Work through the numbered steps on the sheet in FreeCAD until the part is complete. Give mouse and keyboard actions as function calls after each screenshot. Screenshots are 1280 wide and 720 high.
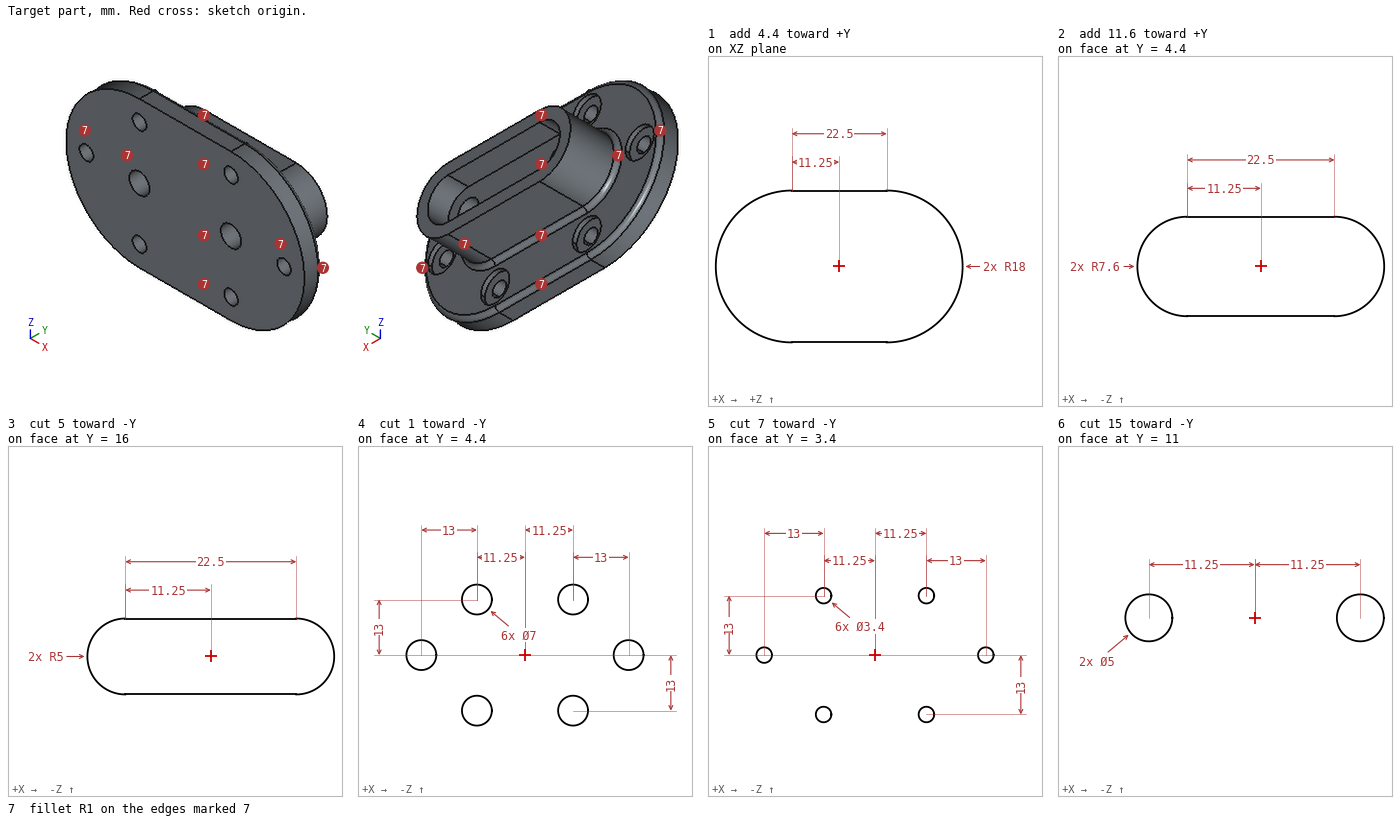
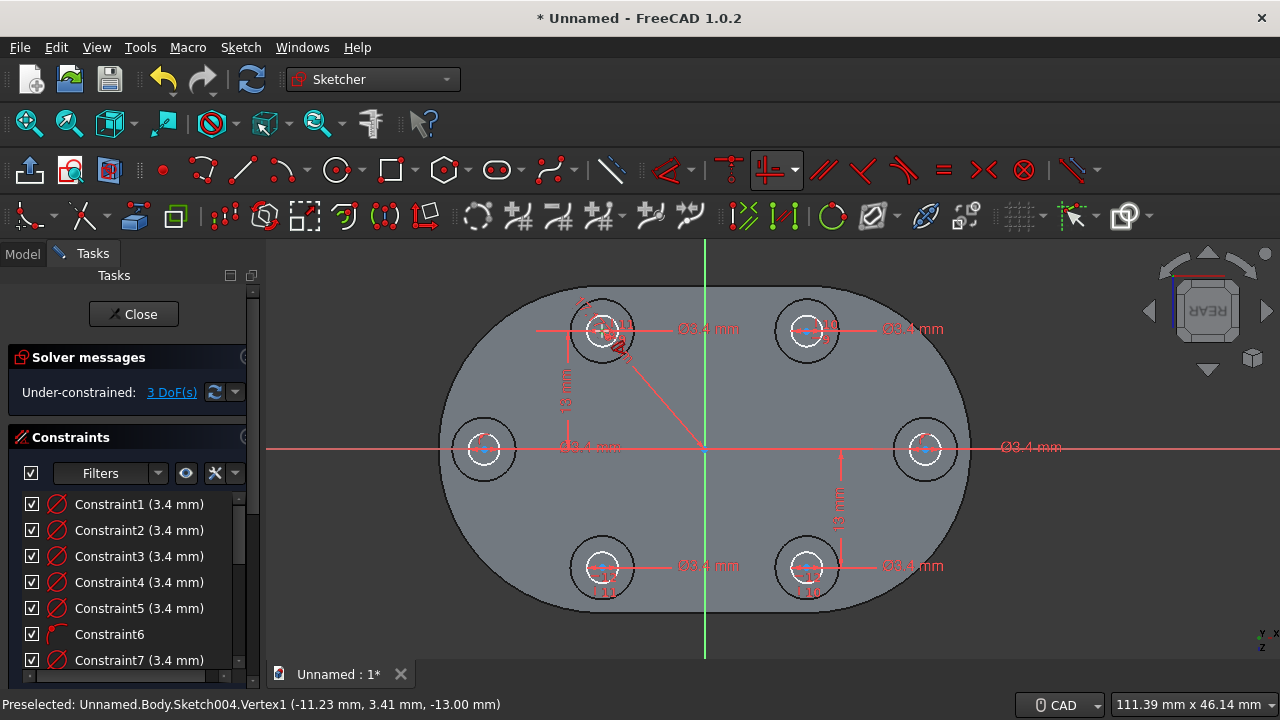
click(484, 449)
click(543, 297)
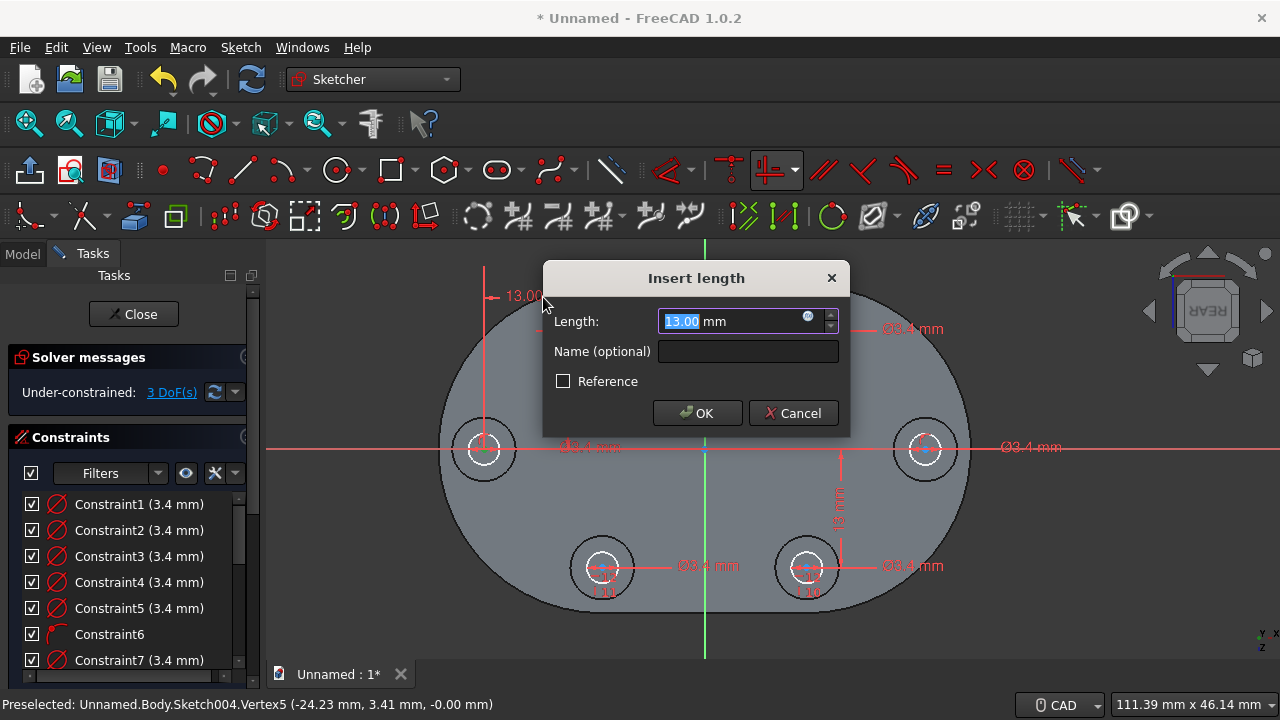
text(13)
key(Return)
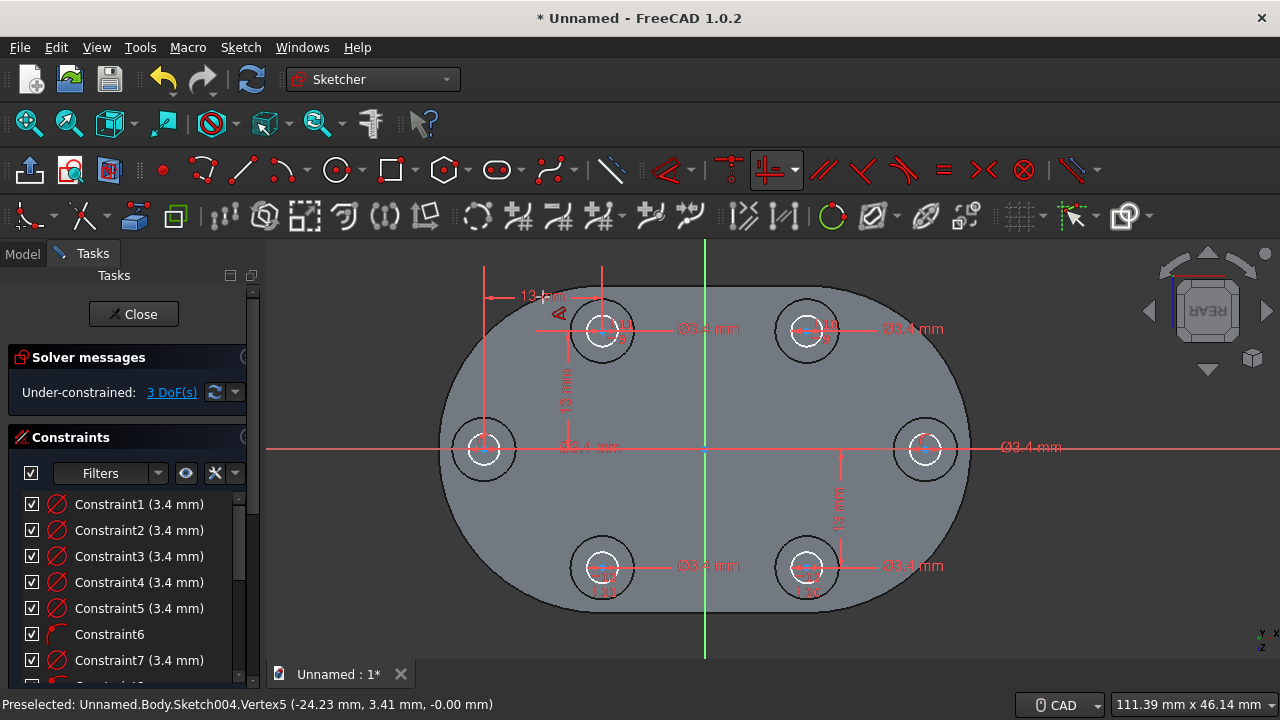
click(807, 331)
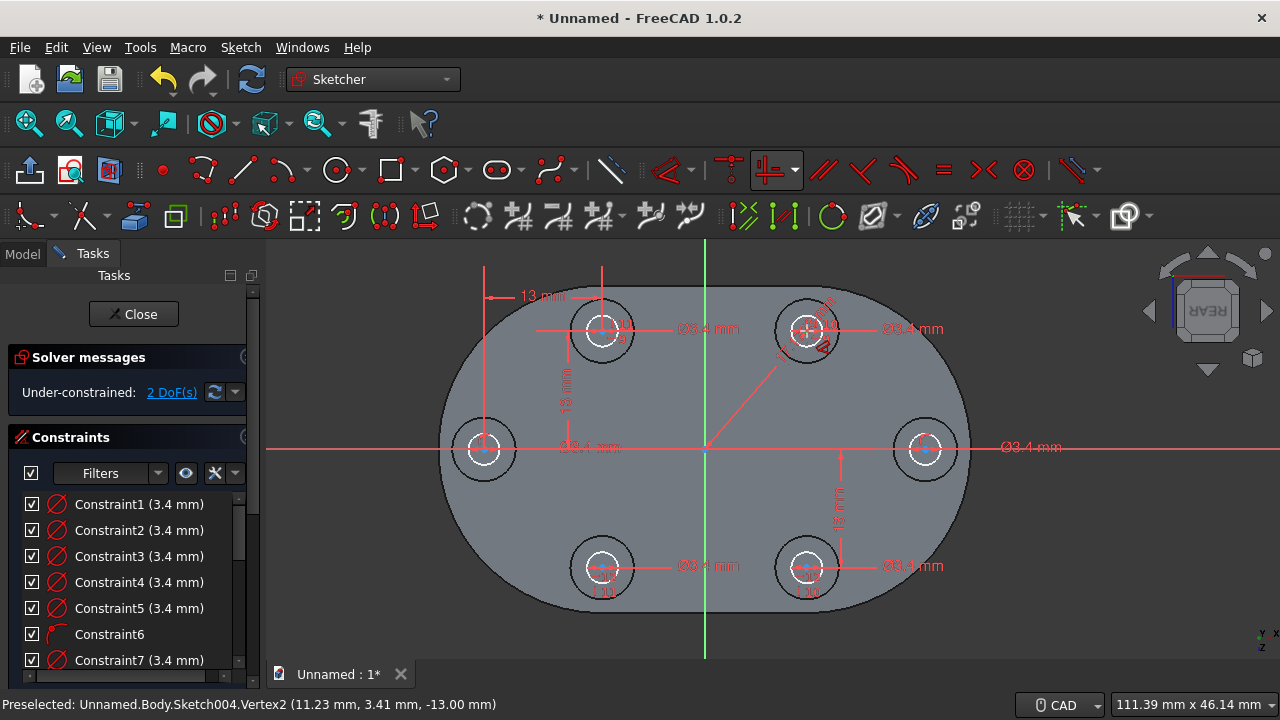
click(925, 449)
click(866, 297)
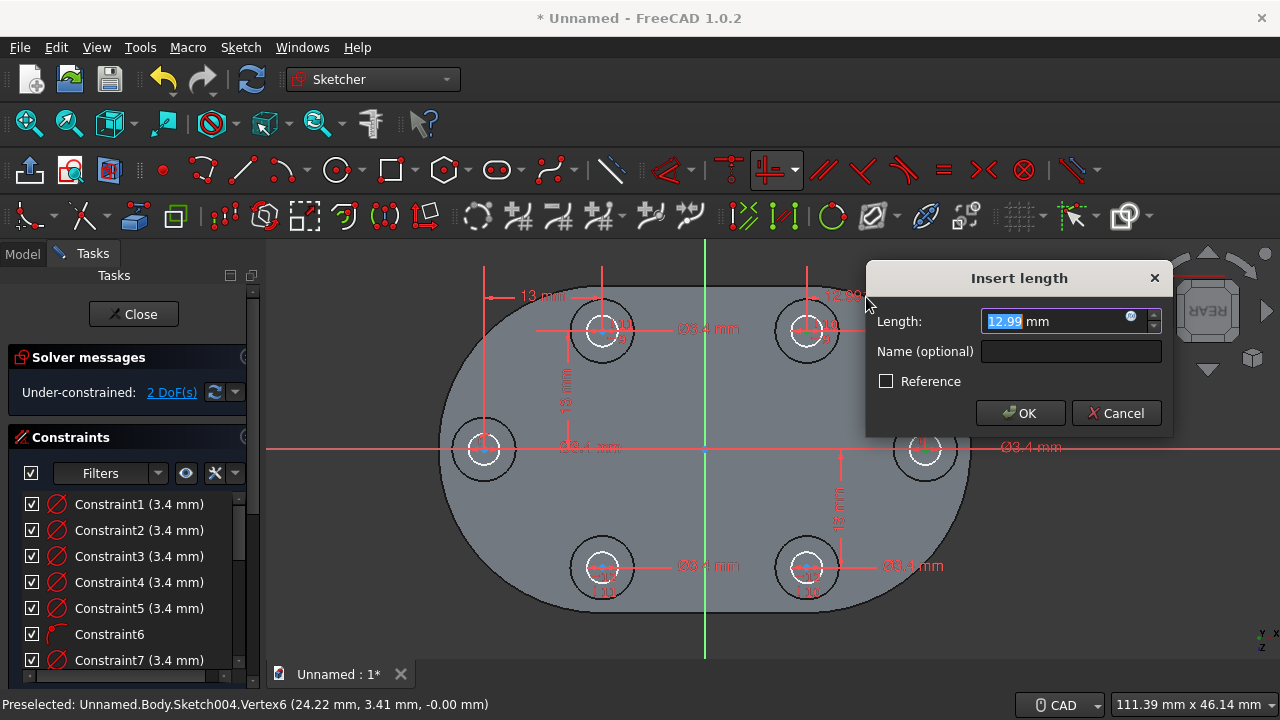
text(13)
key(Return)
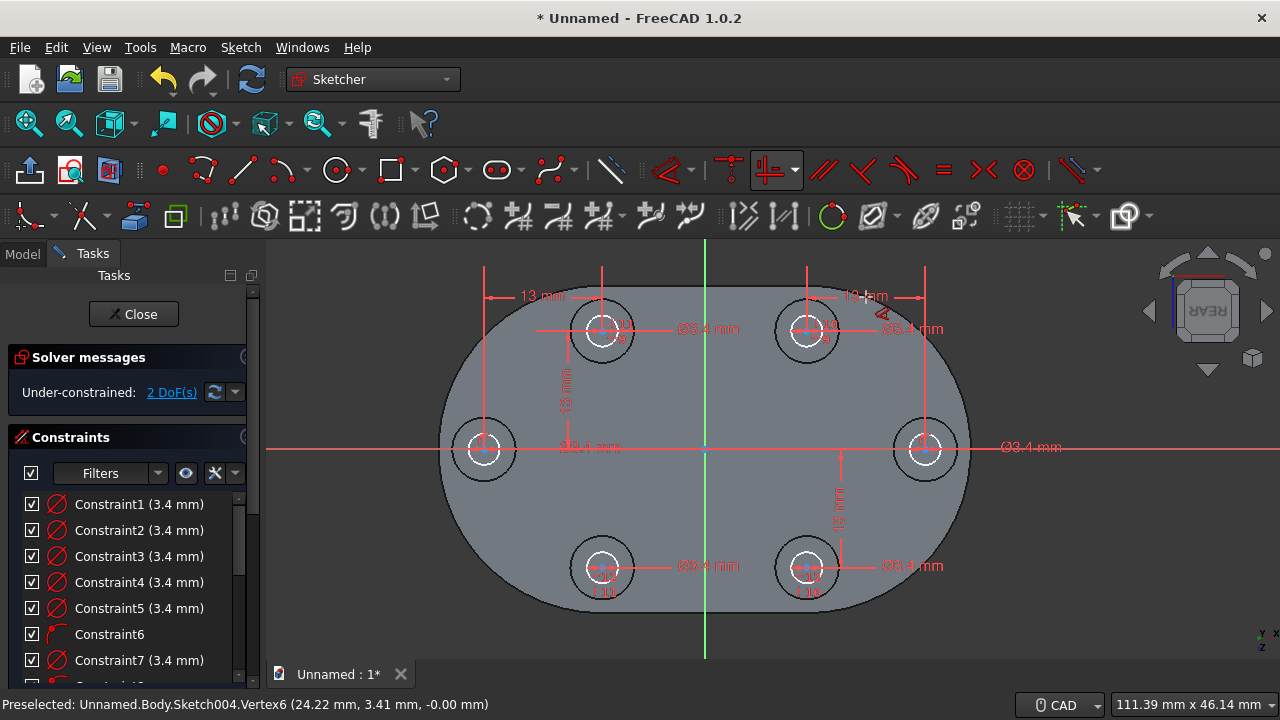
click(602, 331)
click(654, 297)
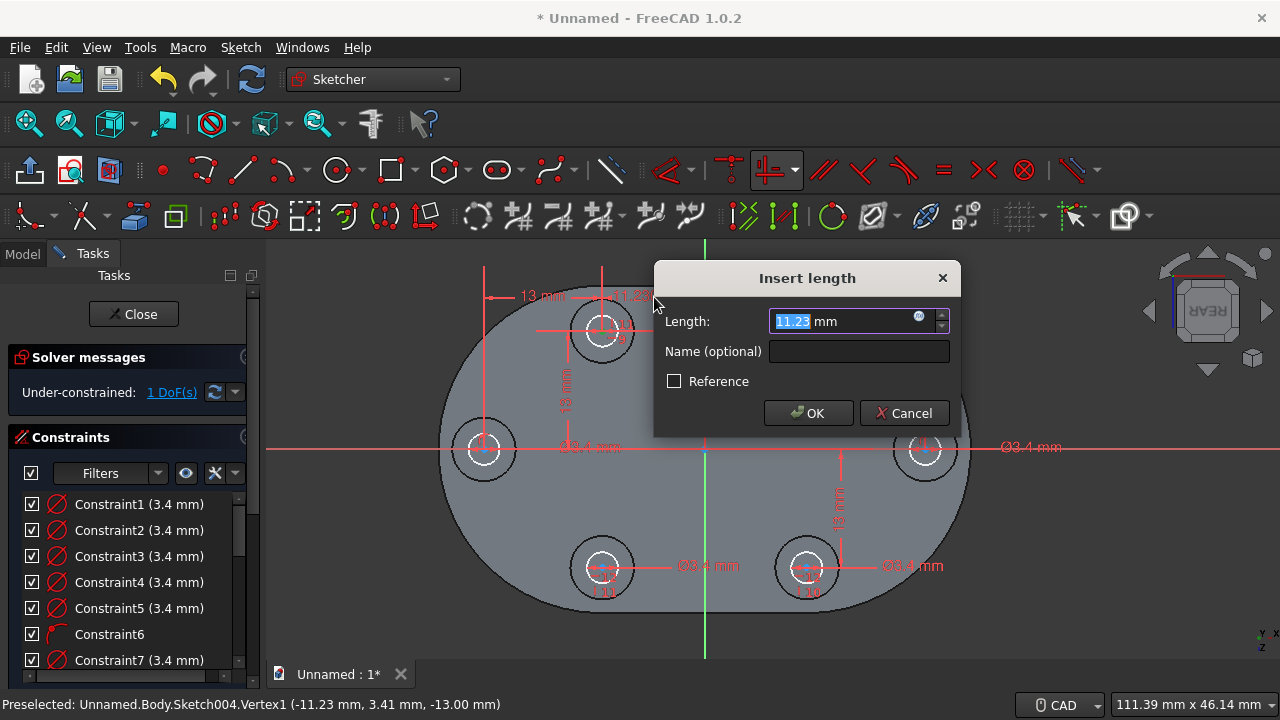
text(11.25)
key(Return)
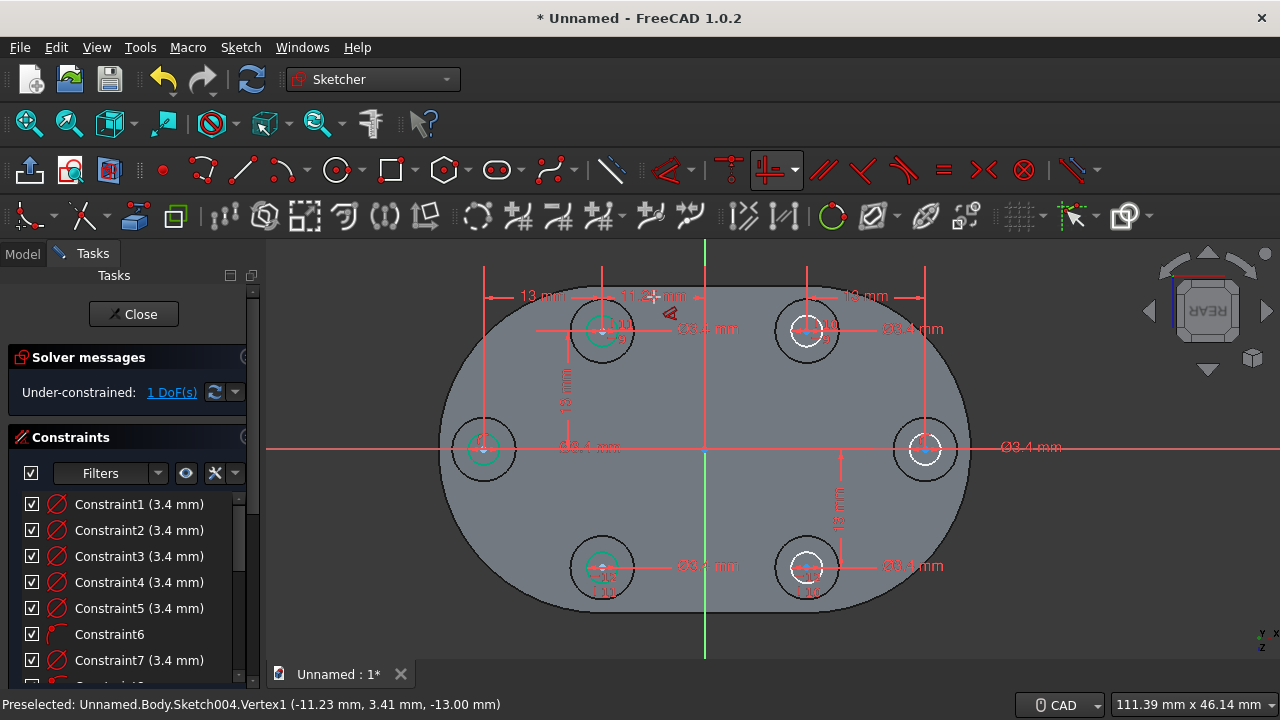
click(807, 331)
click(756, 297)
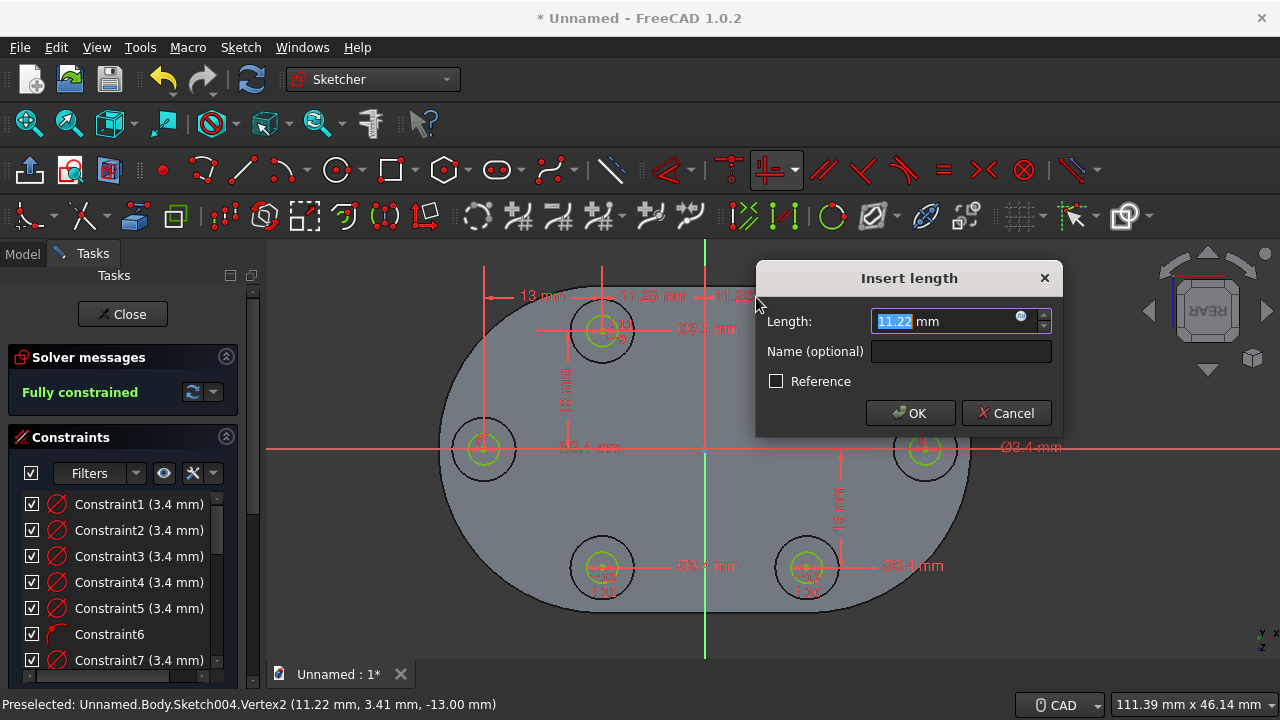
text(11.25)
key(Return)
key(Escape)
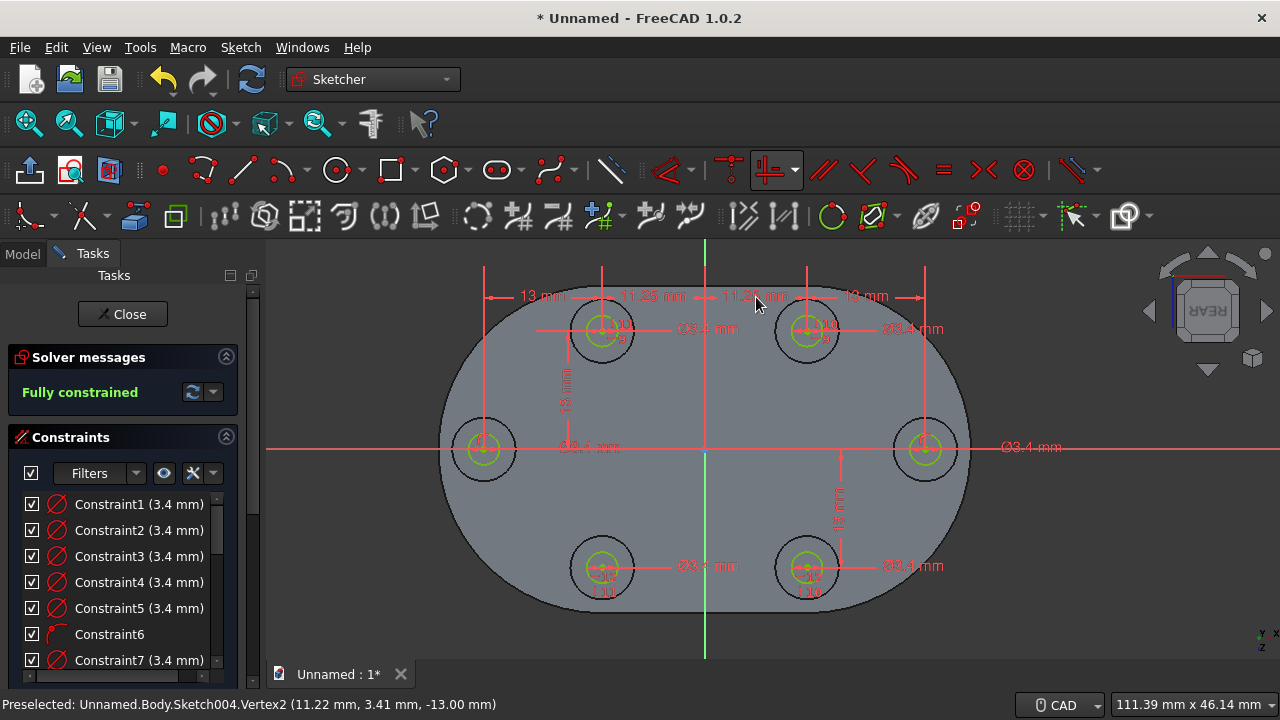
click(123, 314)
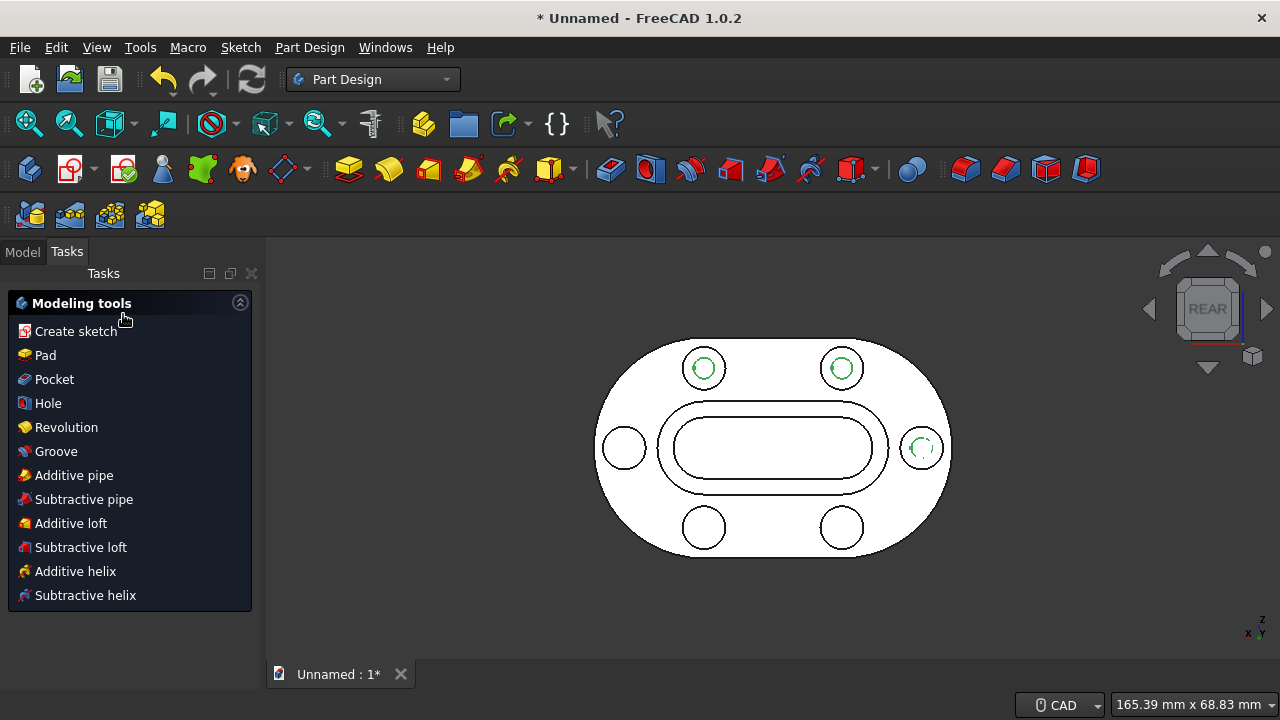
click(612, 170)